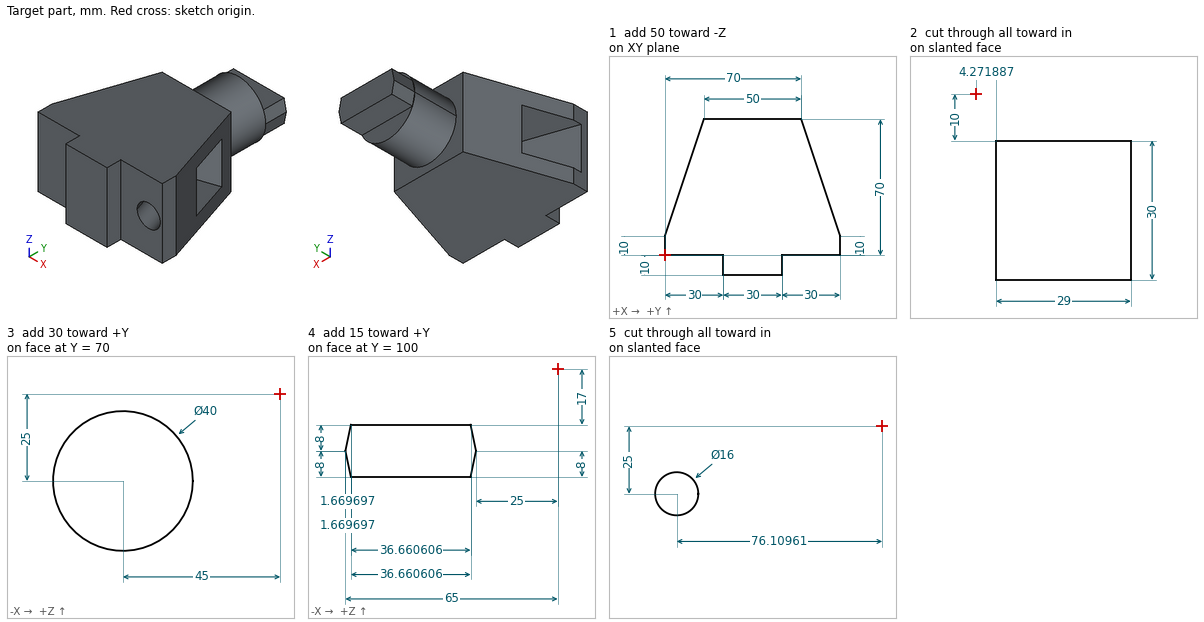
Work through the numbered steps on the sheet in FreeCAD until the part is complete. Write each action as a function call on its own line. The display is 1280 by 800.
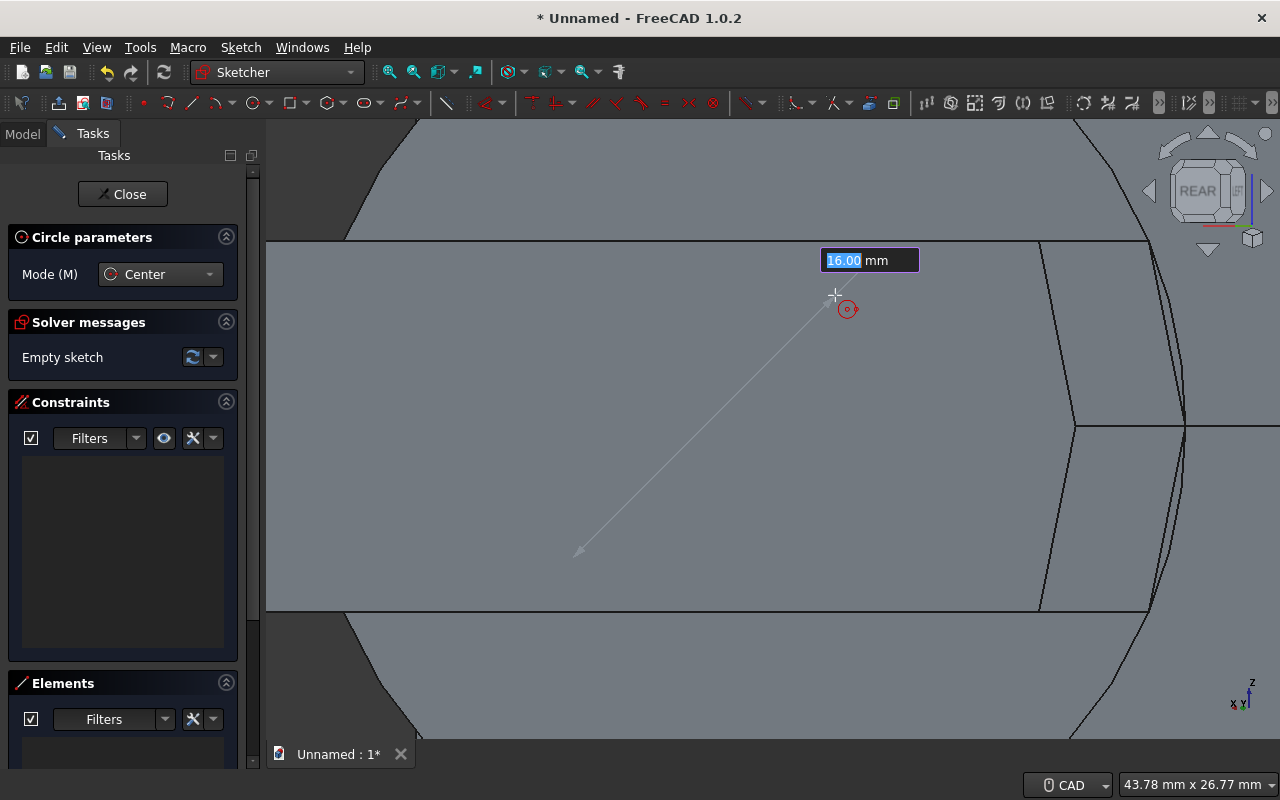
text(16)
key(Return)
key(Escape)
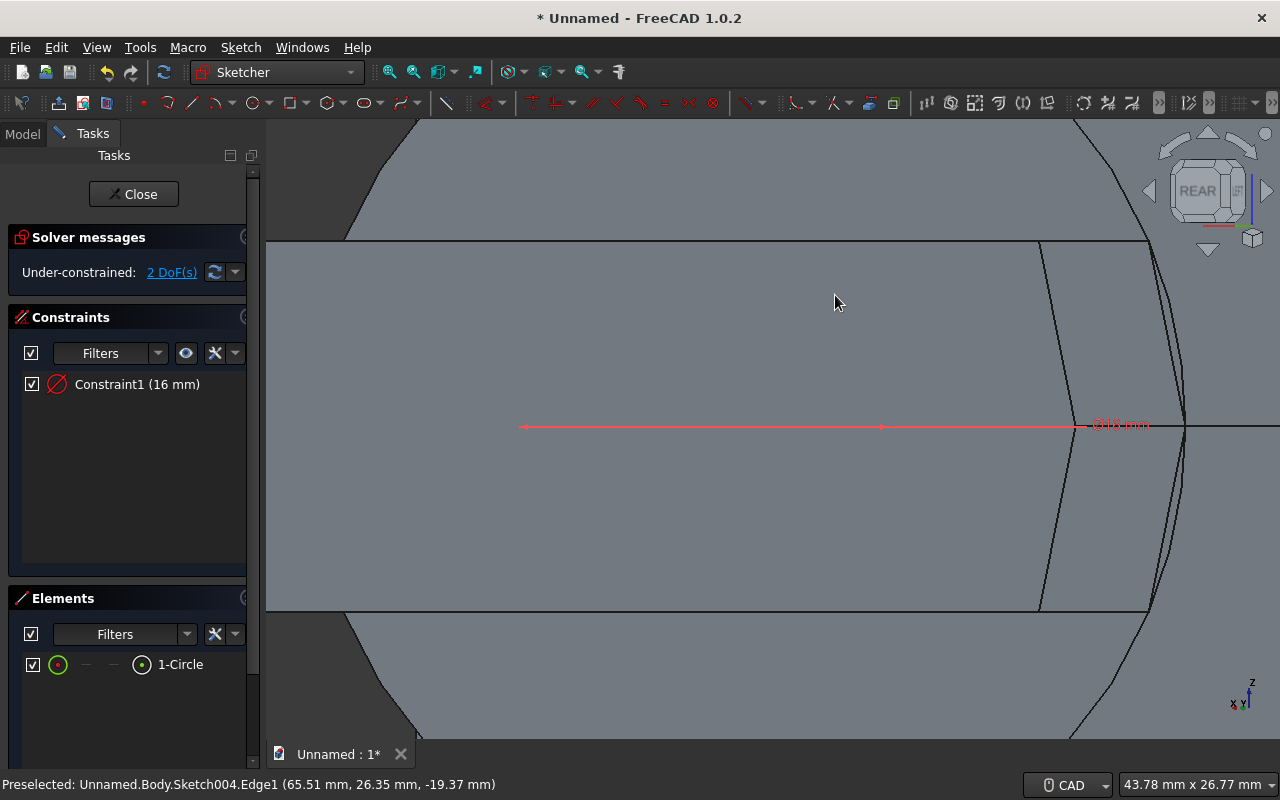
key(d)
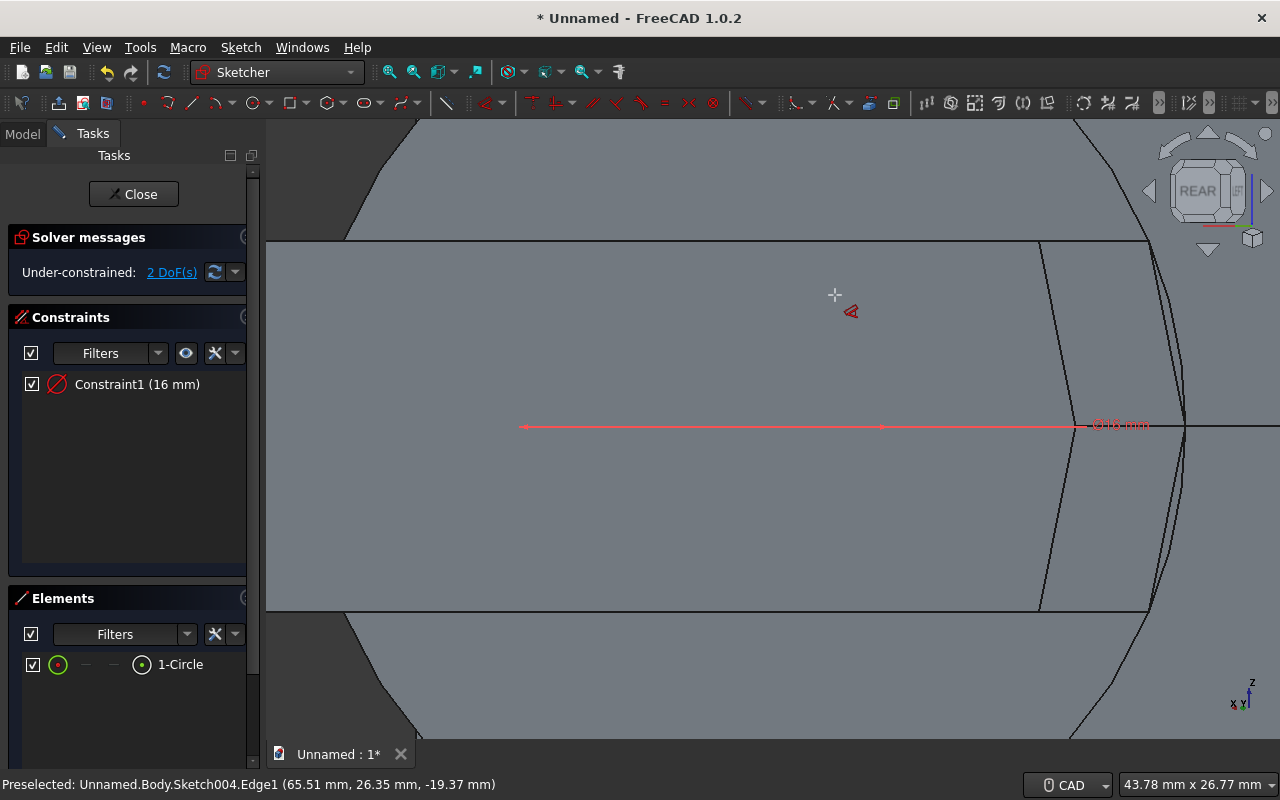
click(704, 427)
click(670, 287)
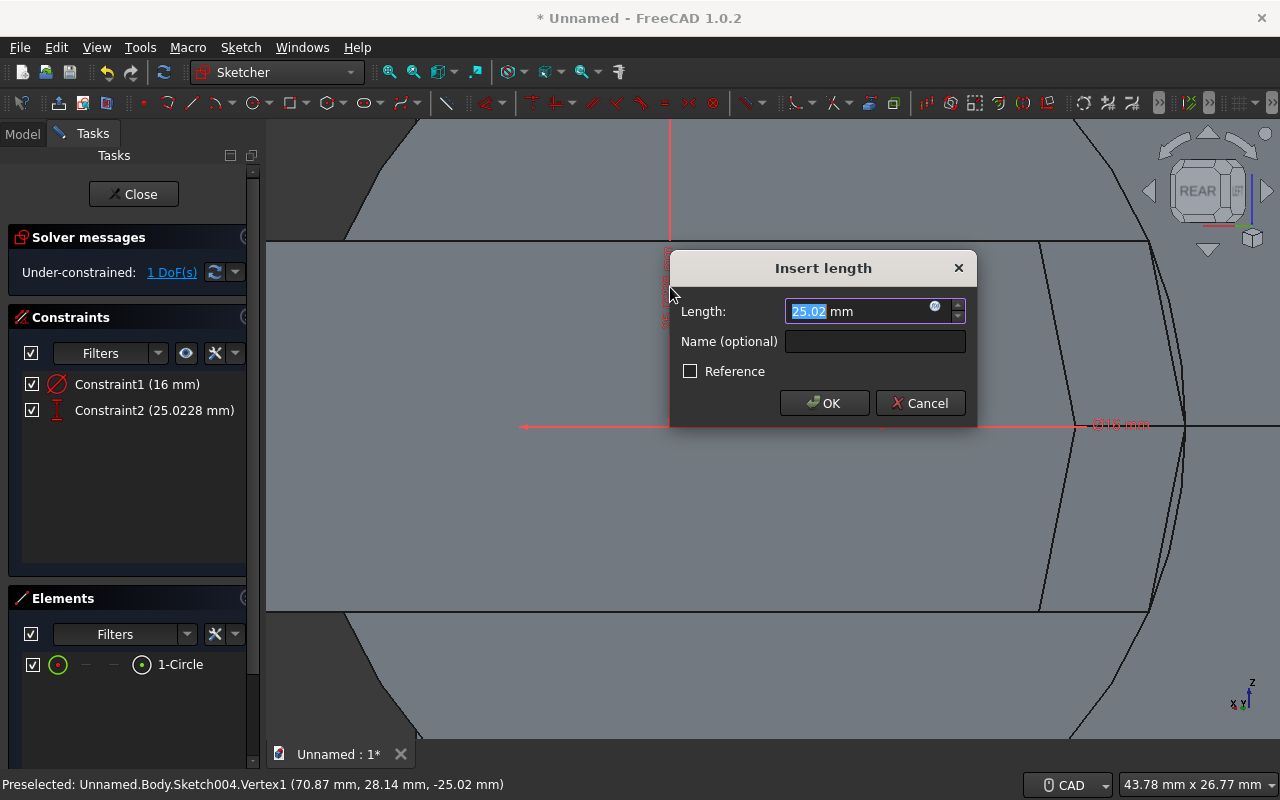
text(25)
key(Return)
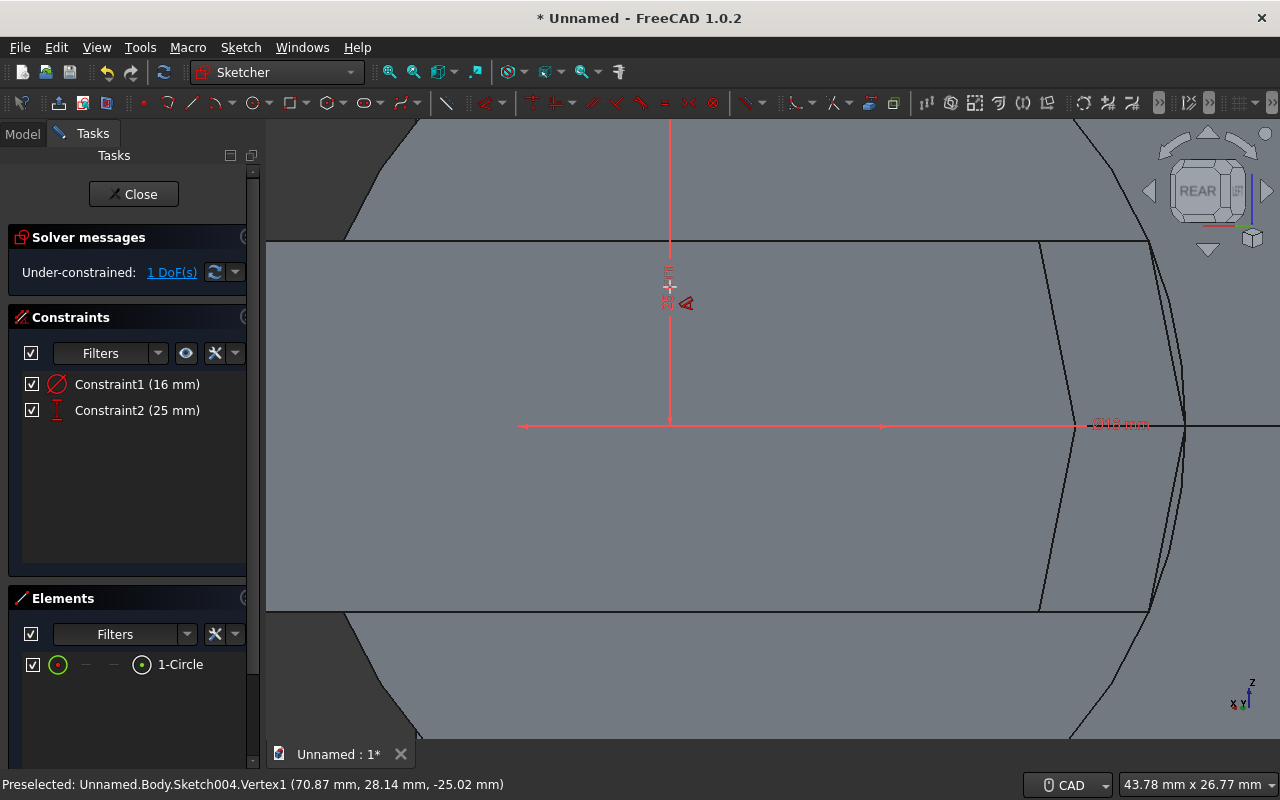
click(704, 426)
click(910, 460)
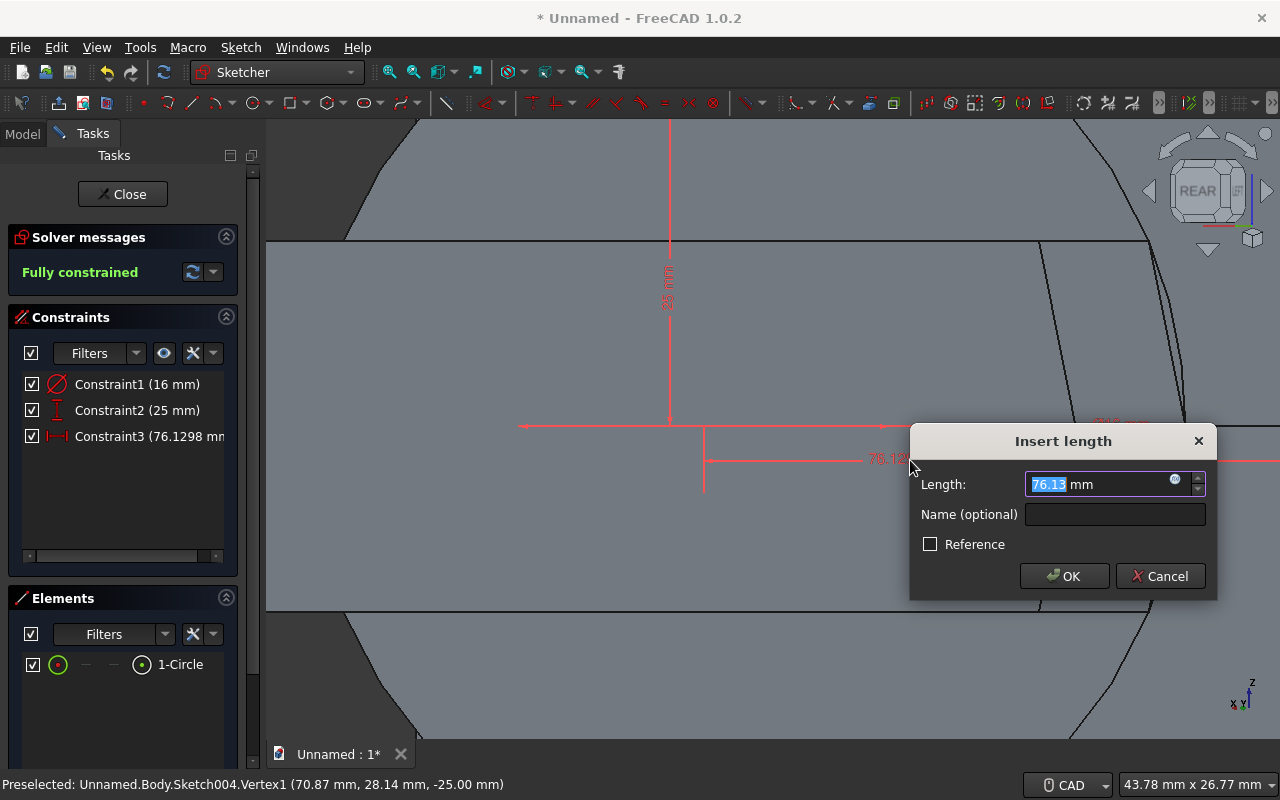
text(76.10961)
key(Return)
key(Escape)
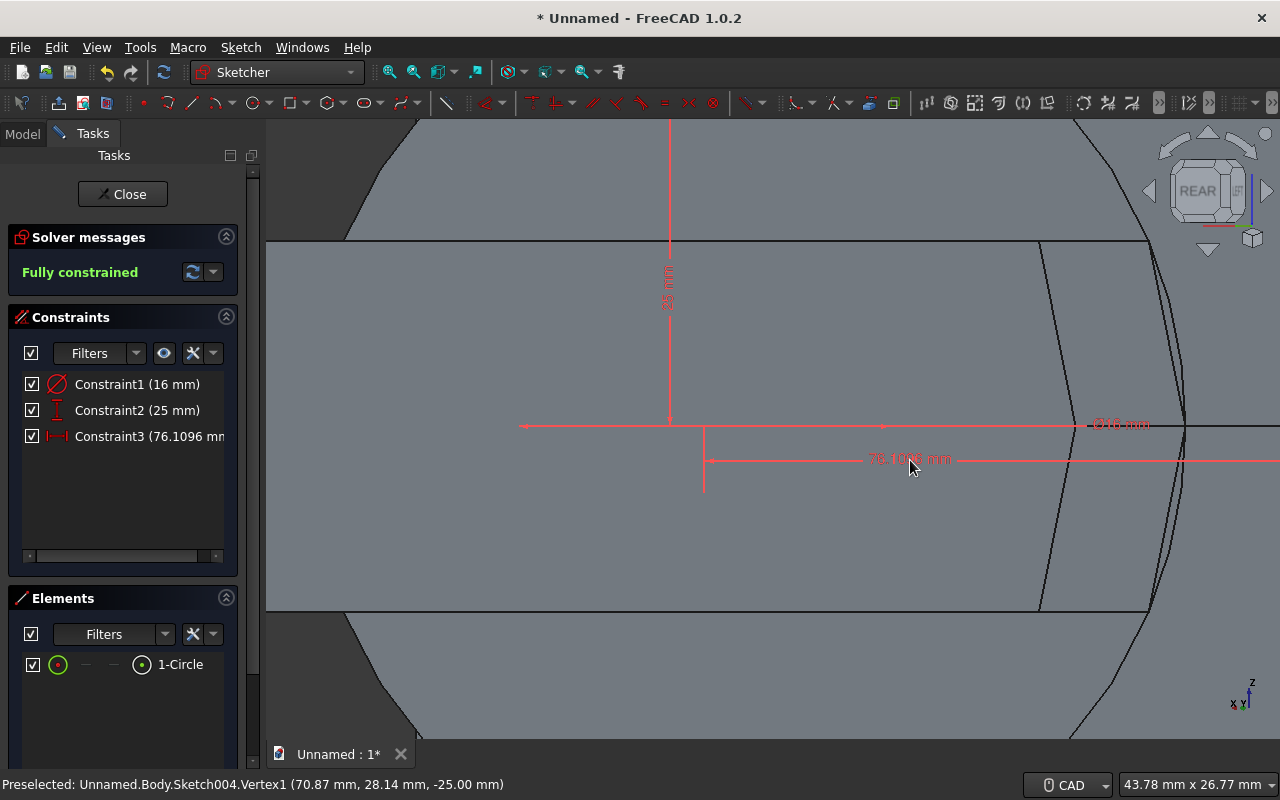
click(123, 194)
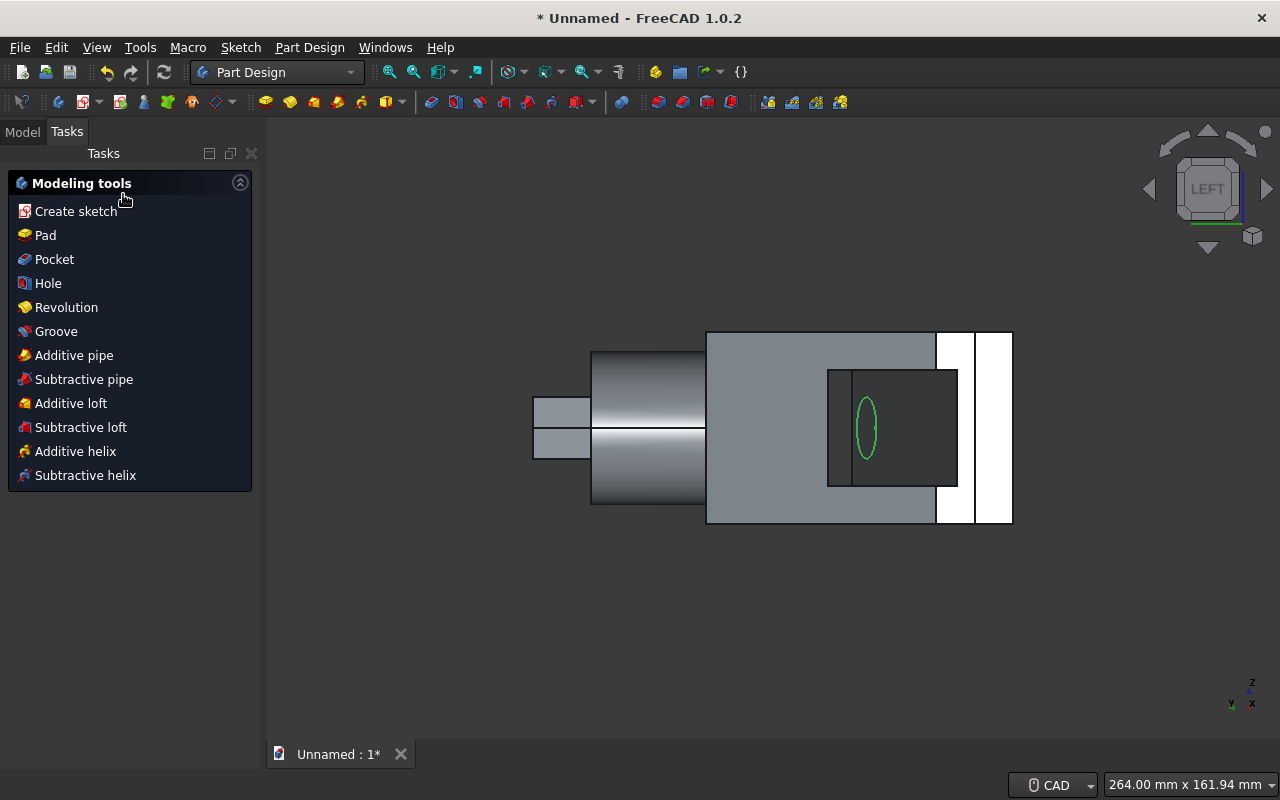
click(432, 102)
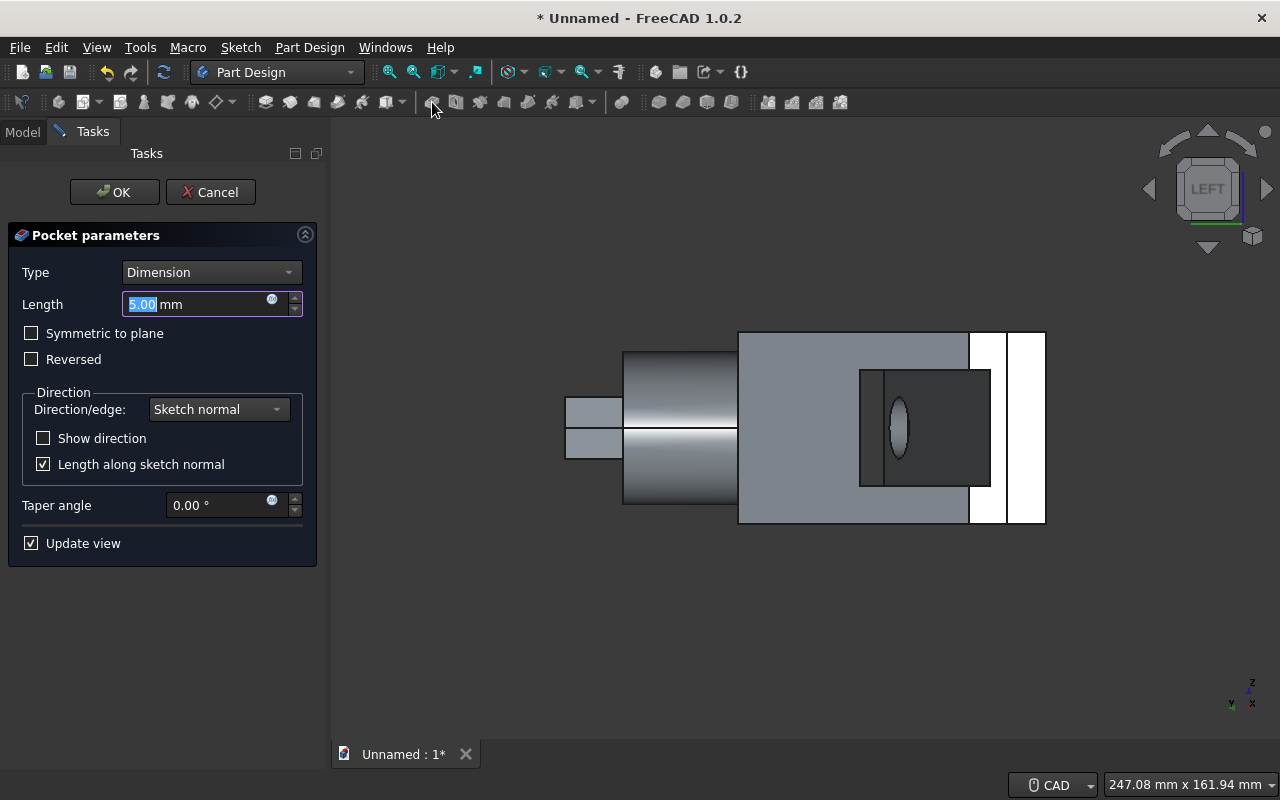
click(212, 272)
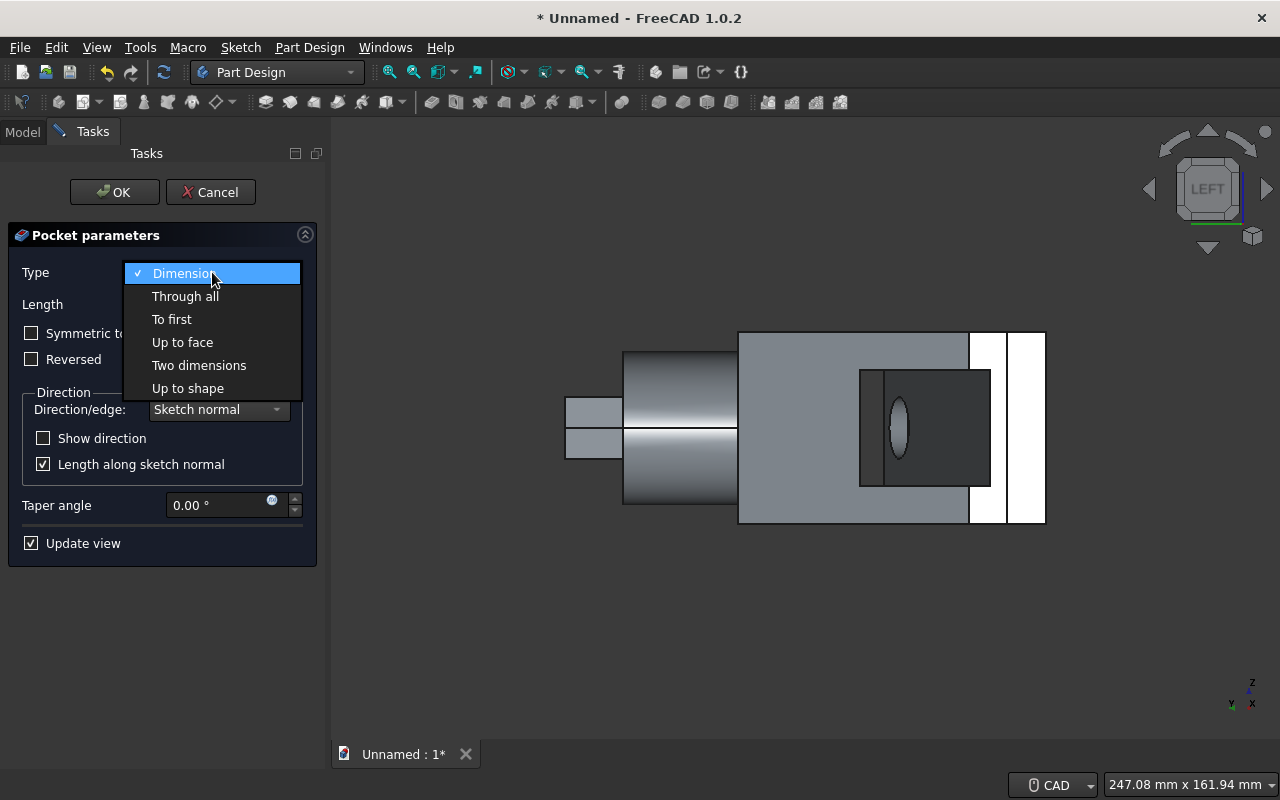
click(212, 296)